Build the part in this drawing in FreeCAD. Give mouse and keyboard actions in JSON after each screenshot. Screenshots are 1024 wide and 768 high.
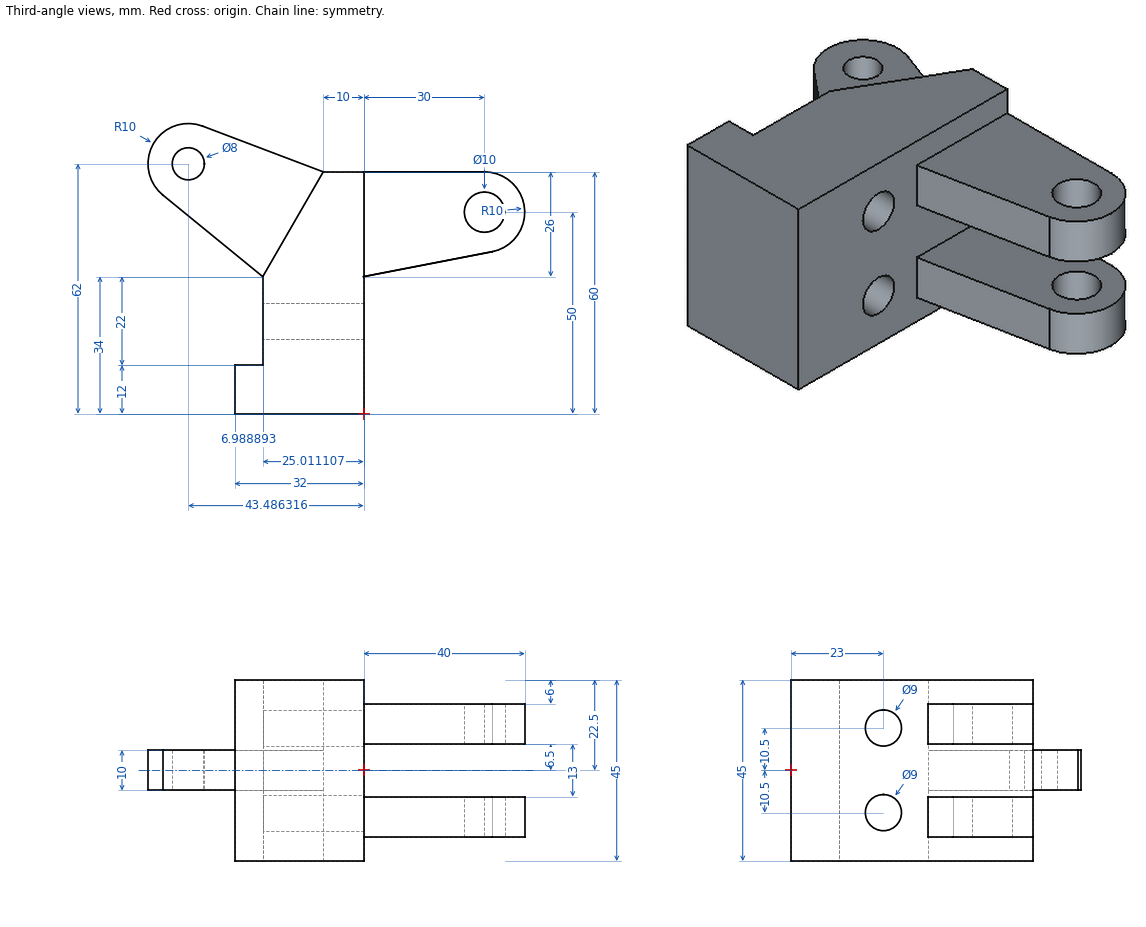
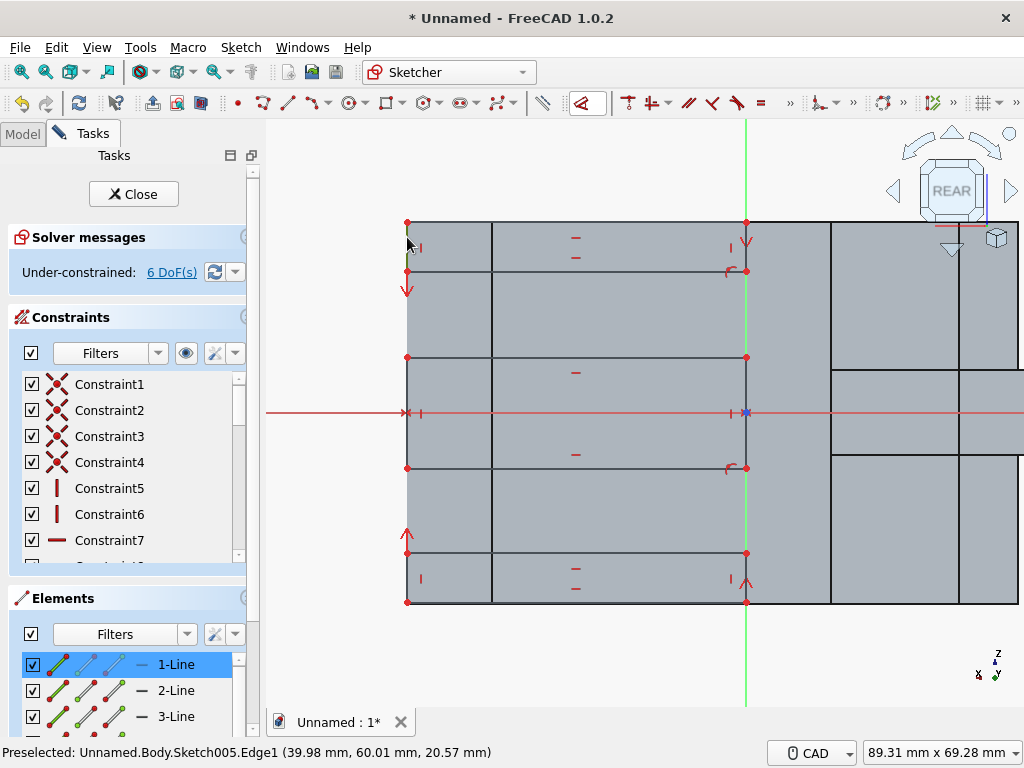
{"action": "key", "text": "i"}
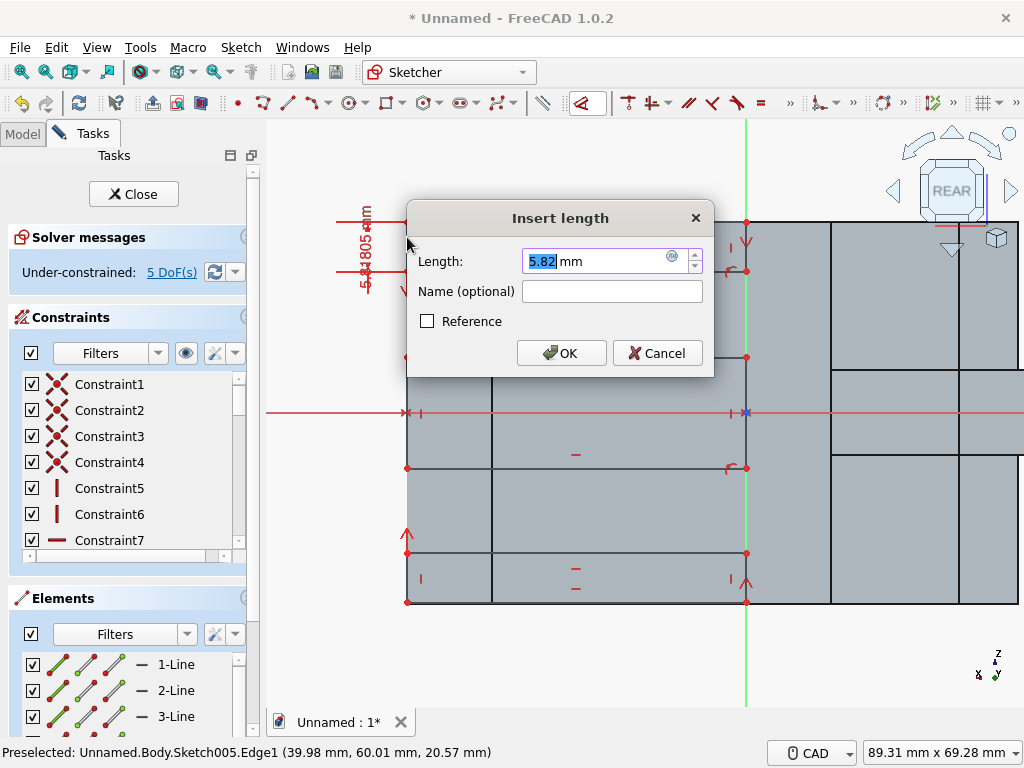
{"action": "type", "text": "6"}
{"action": "key", "text": "Return"}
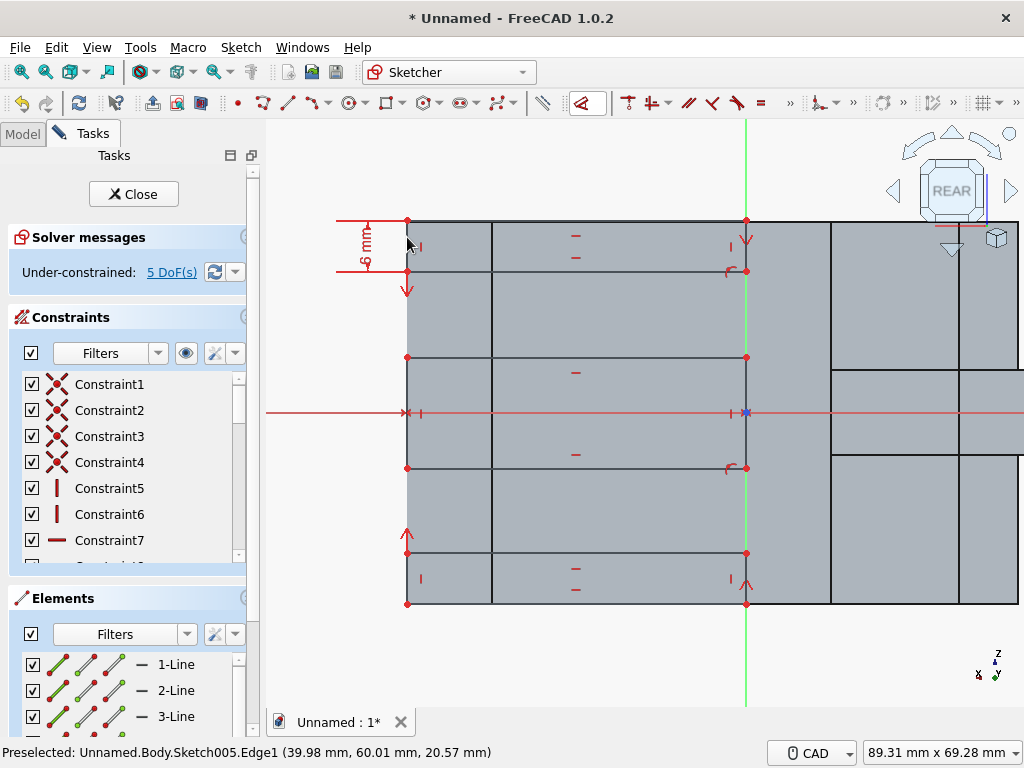
{"action": "left_click", "coordinate": [509, 272]}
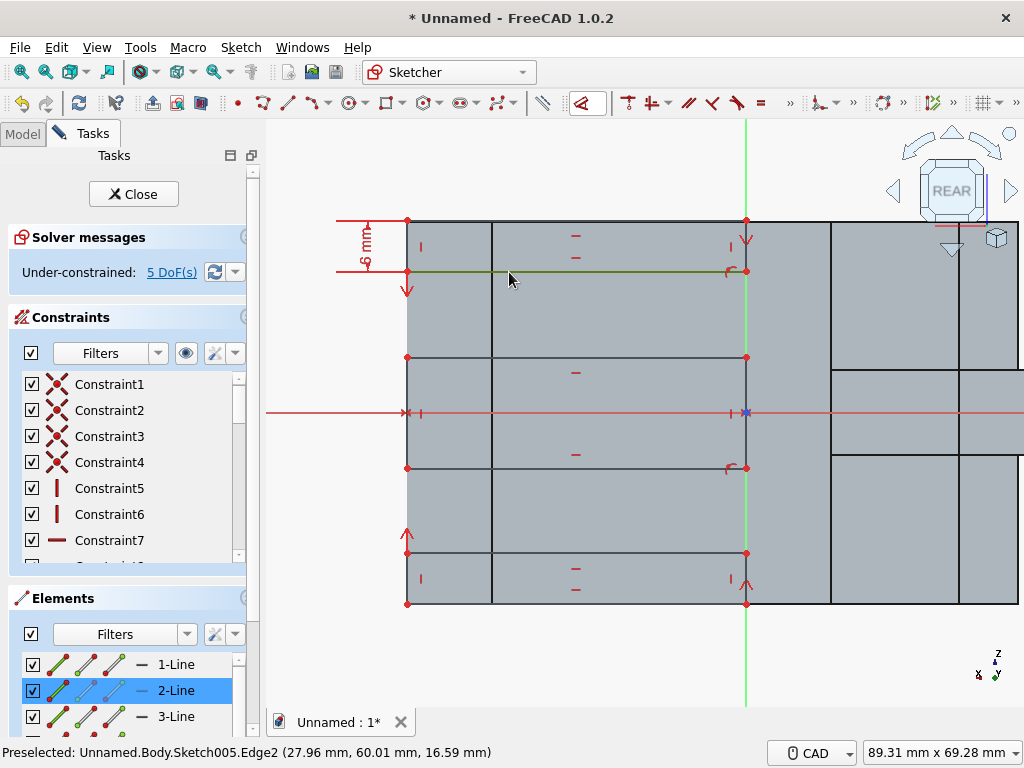
{"action": "left_click", "coordinate": [600, 104]}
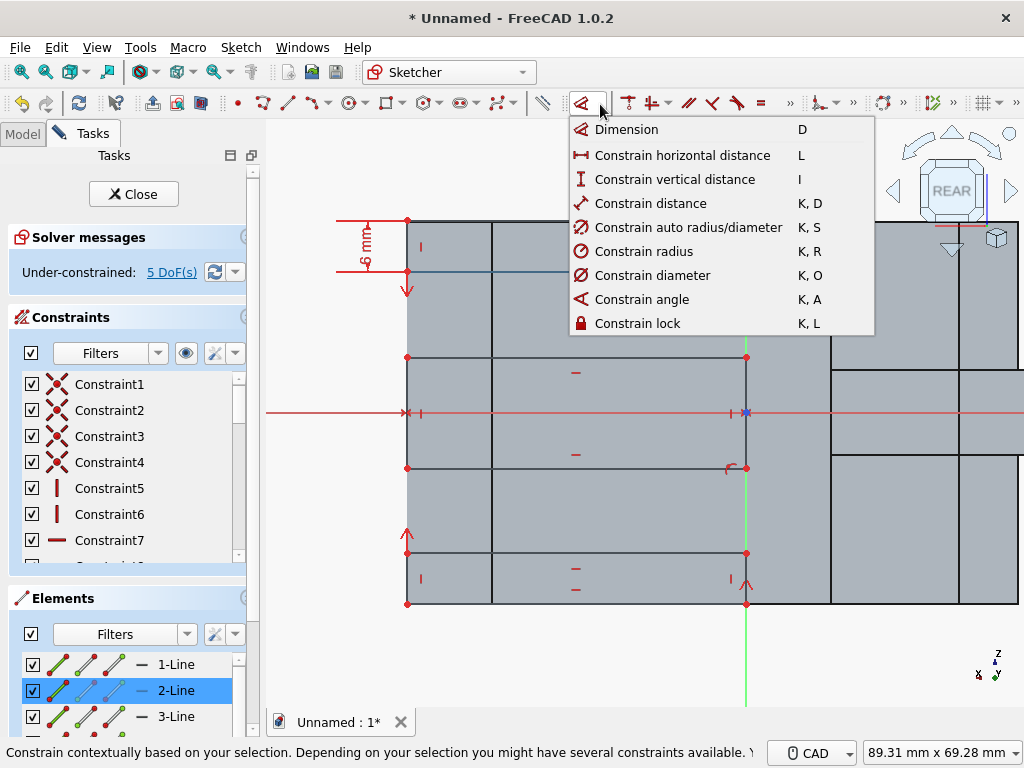
{"action": "left_click", "coordinate": [722, 155]}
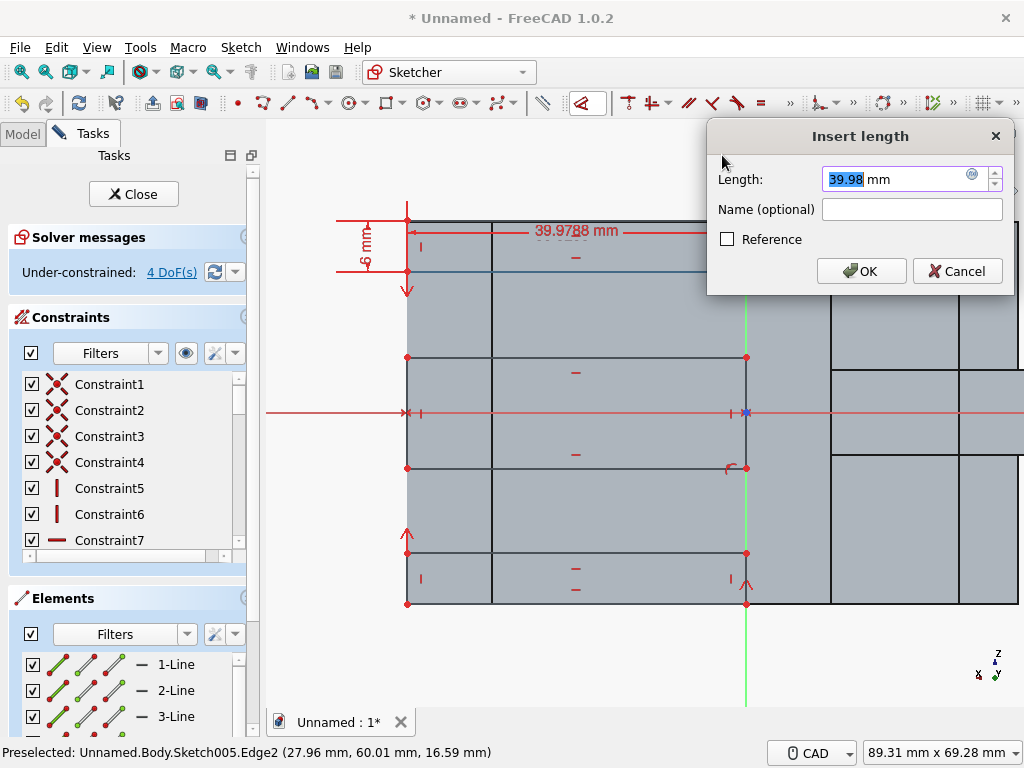
{"action": "type", "text": "40"}
{"action": "key", "text": "Return"}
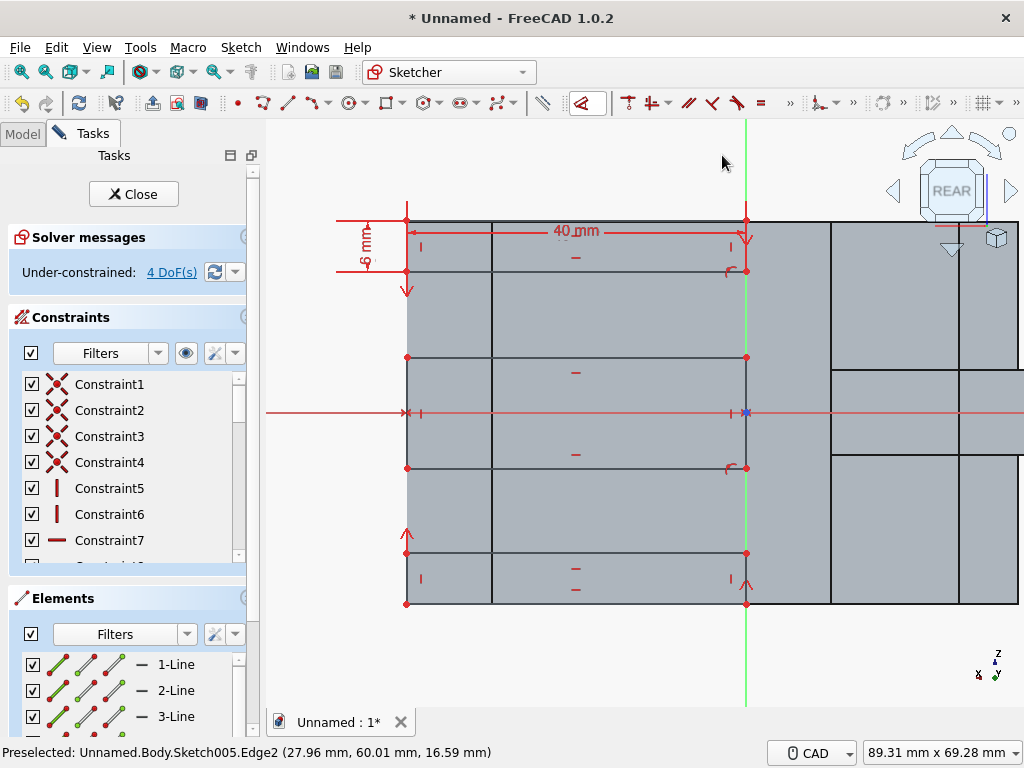
{"action": "left_click", "coordinate": [407, 391]}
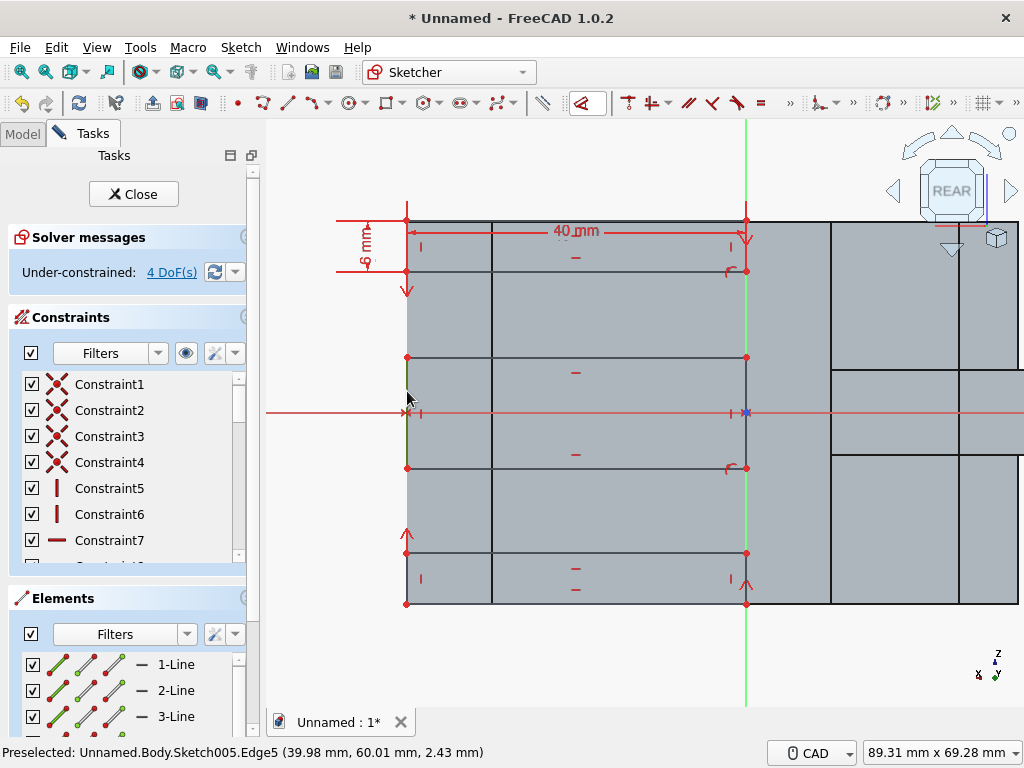
{"action": "key", "text": "i"}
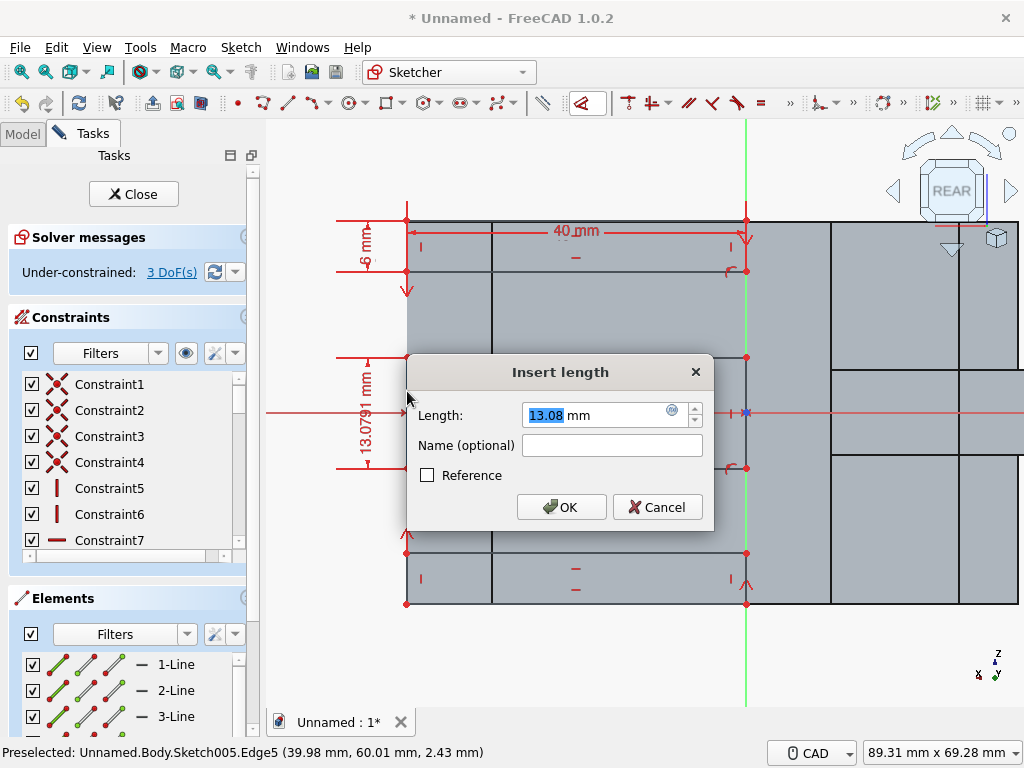
{"action": "type", "text": "13"}
{"action": "key", "text": "Return"}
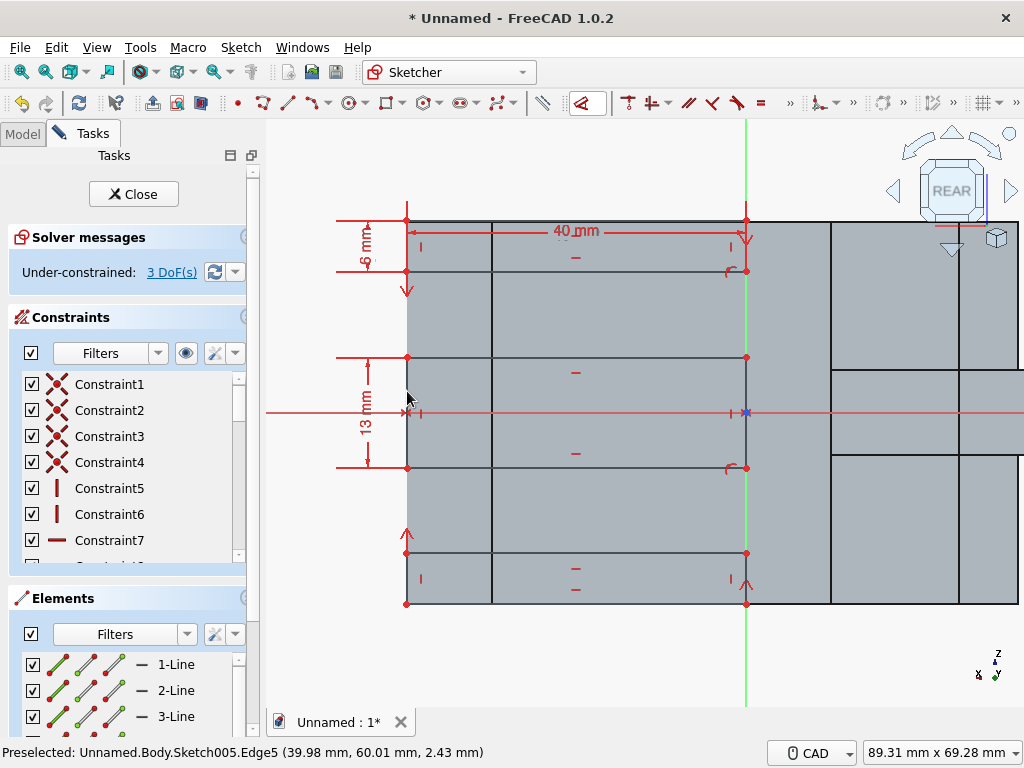
{"action": "left_click", "coordinate": [509, 468]}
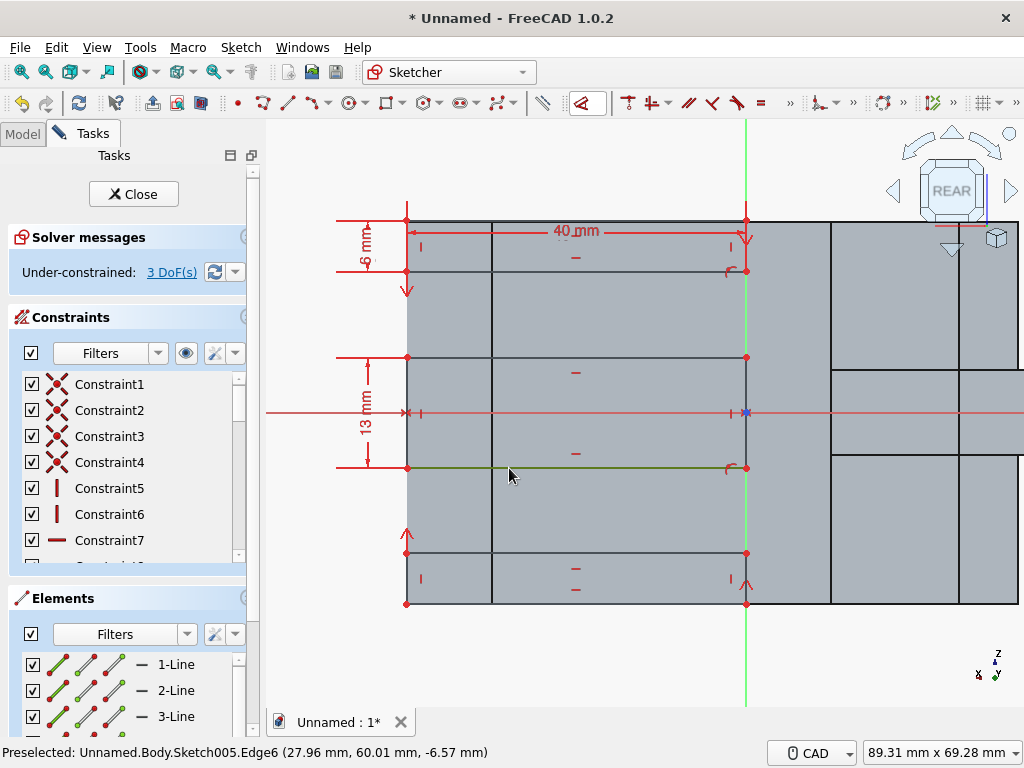
{"action": "key", "text": "l"}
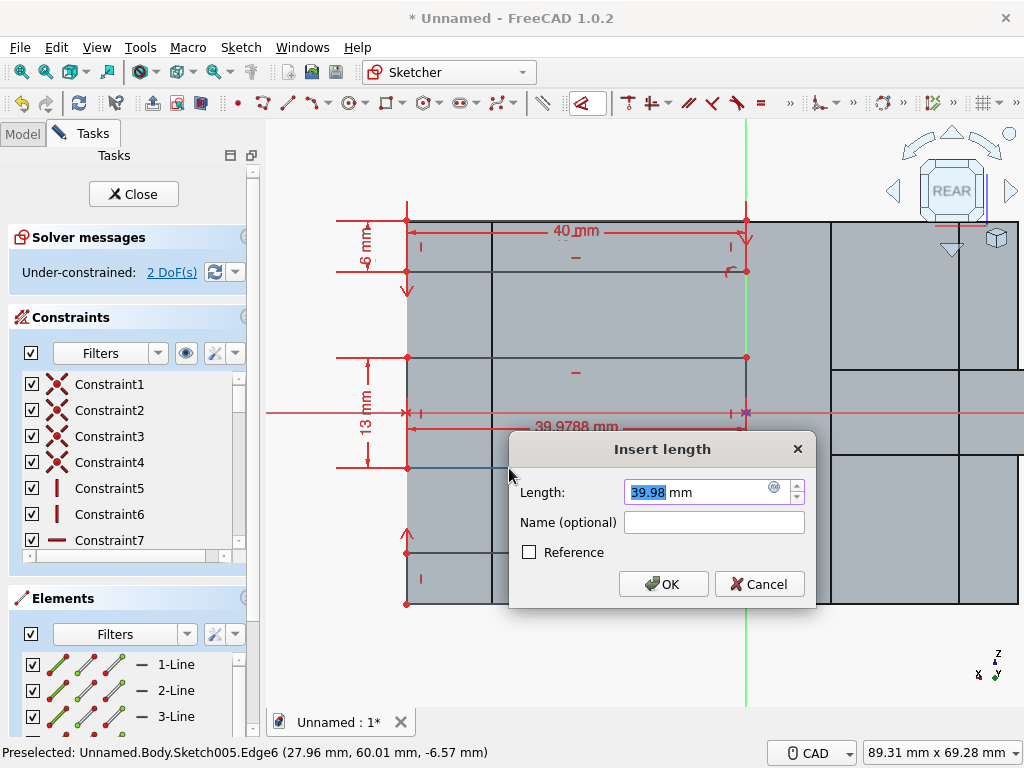
{"action": "type", "text": "40"}
{"action": "key", "text": "Return"}